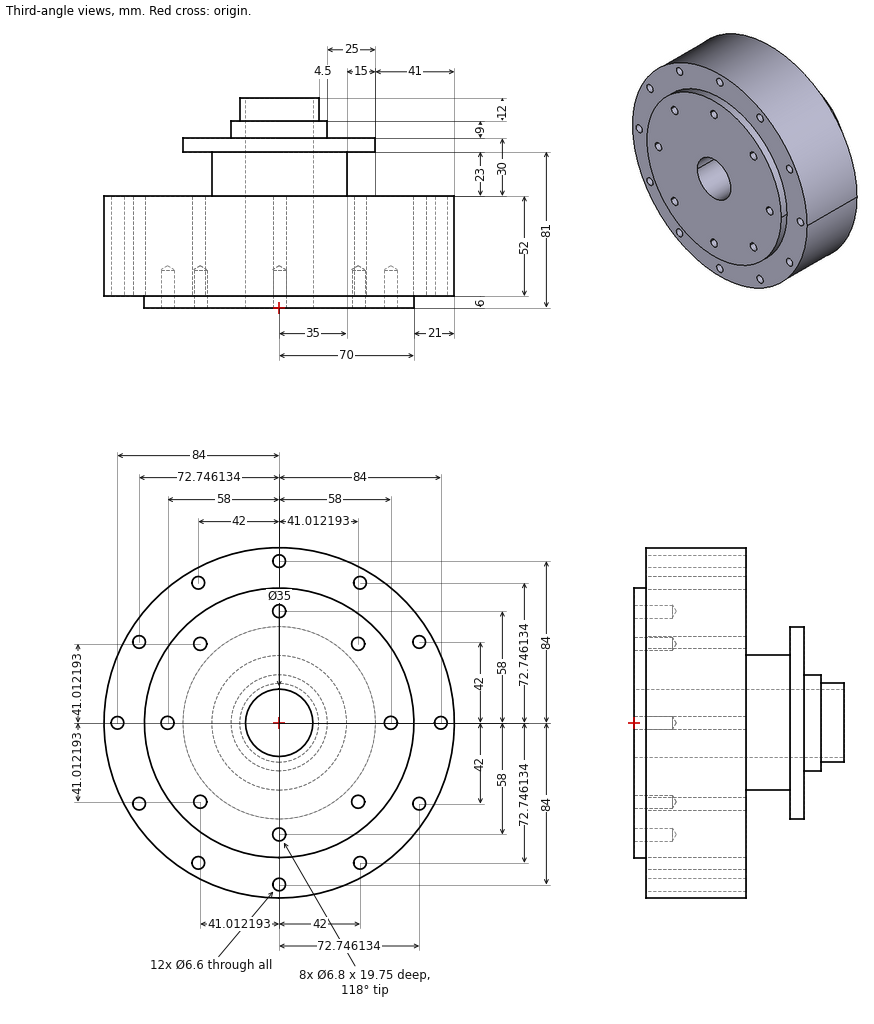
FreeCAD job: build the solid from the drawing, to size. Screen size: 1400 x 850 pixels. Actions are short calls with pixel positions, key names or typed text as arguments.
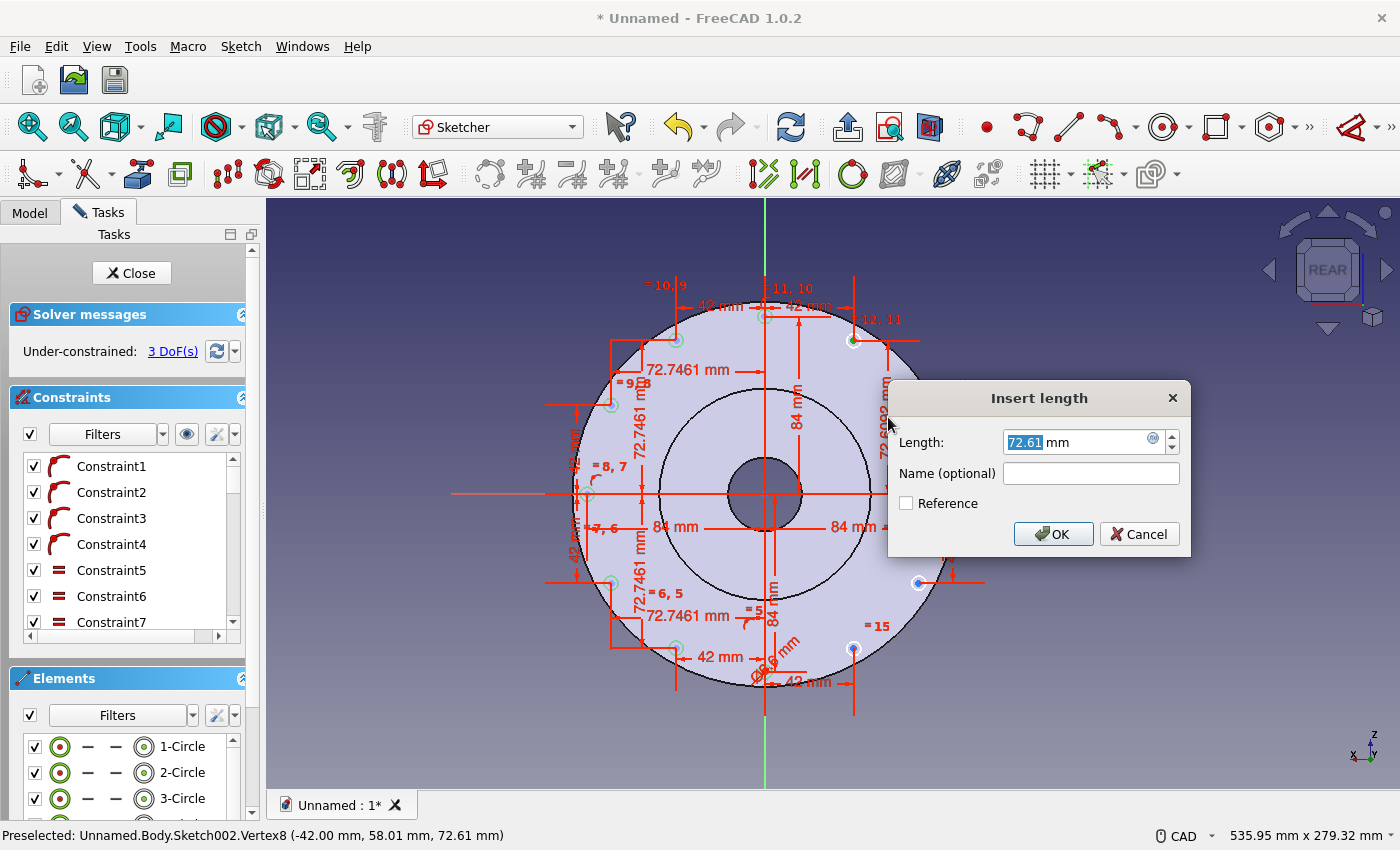
text(72.746134)
key(Return)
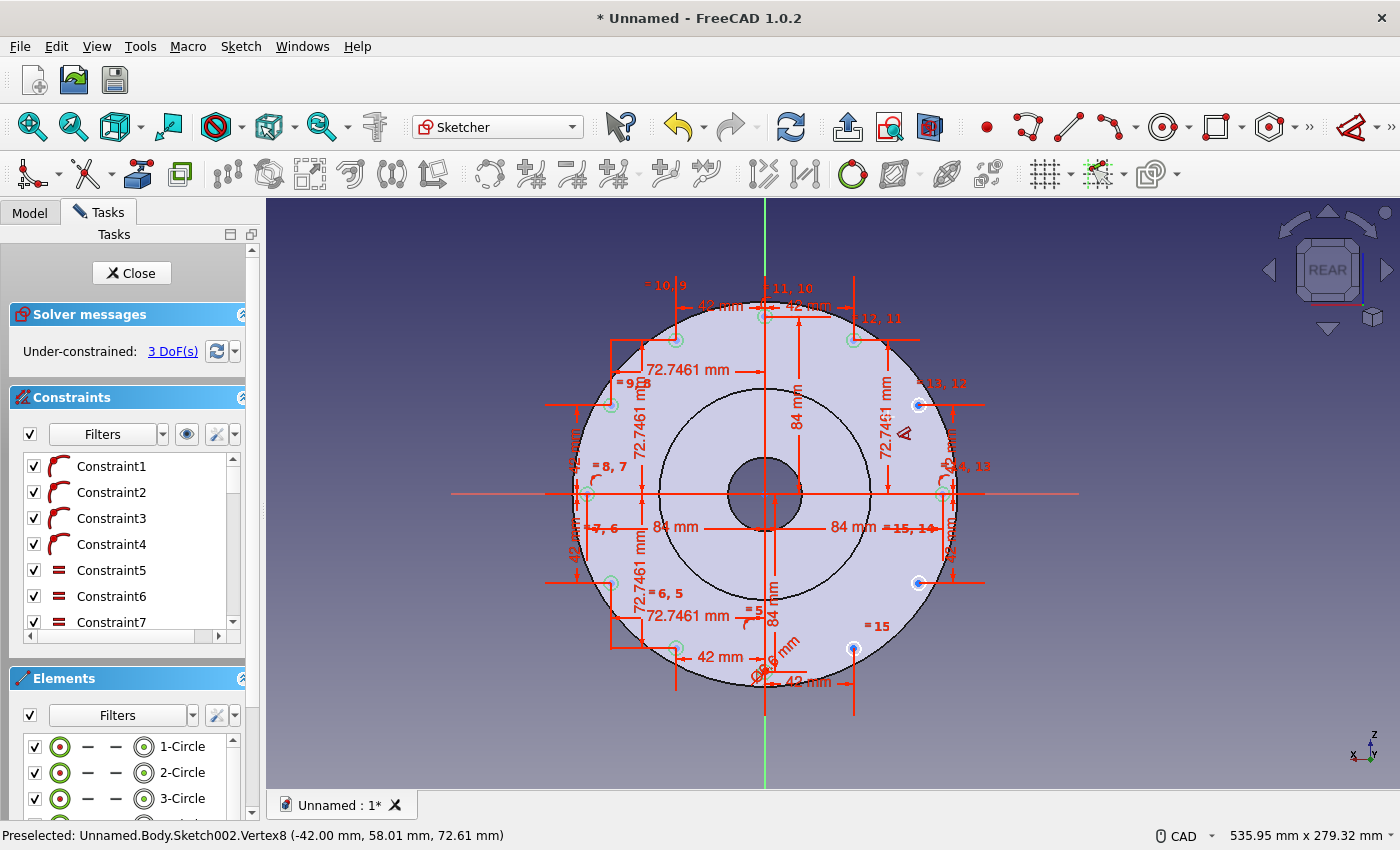
click(919, 405)
click(842, 371)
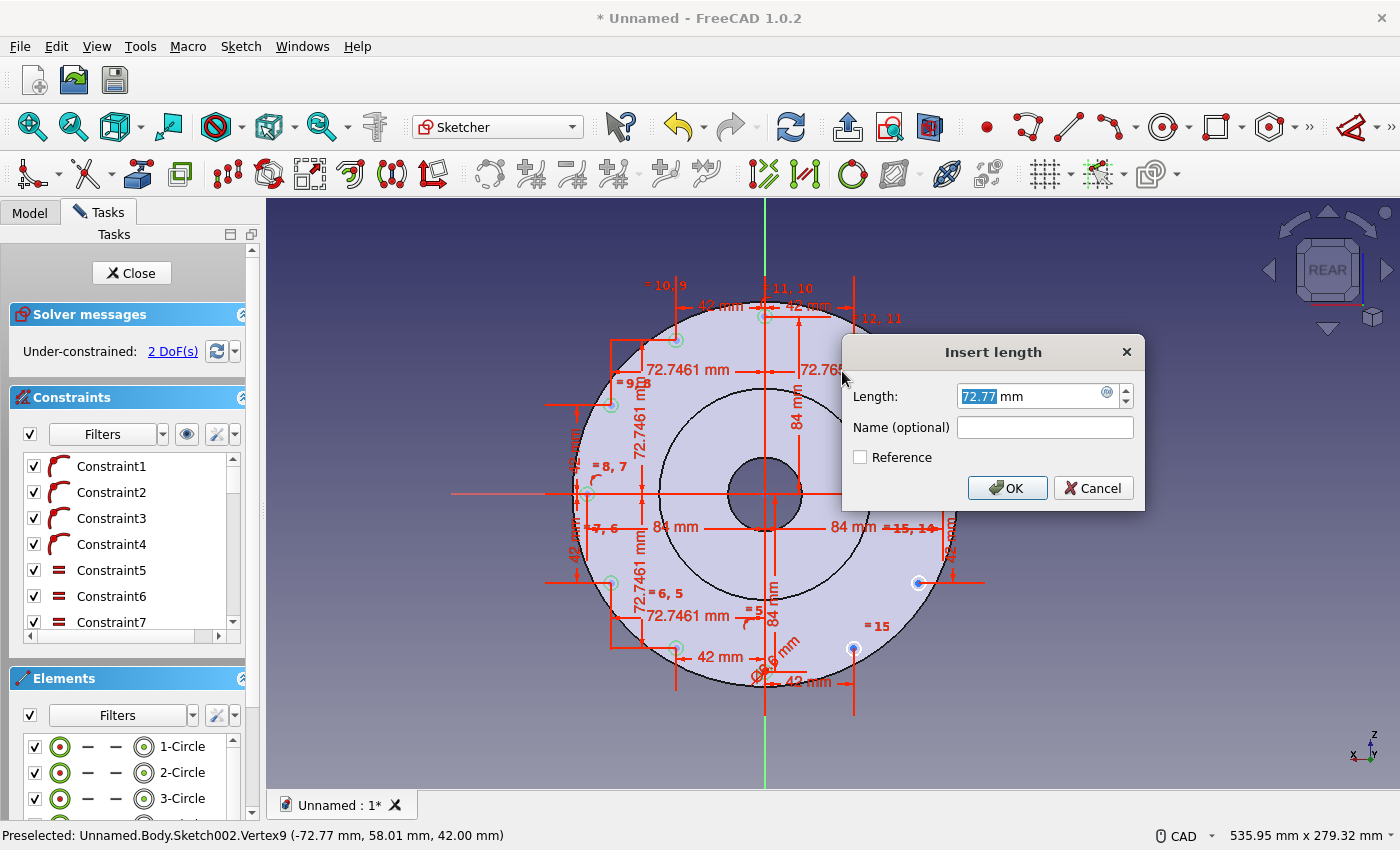
text(72.746134)
key(Return)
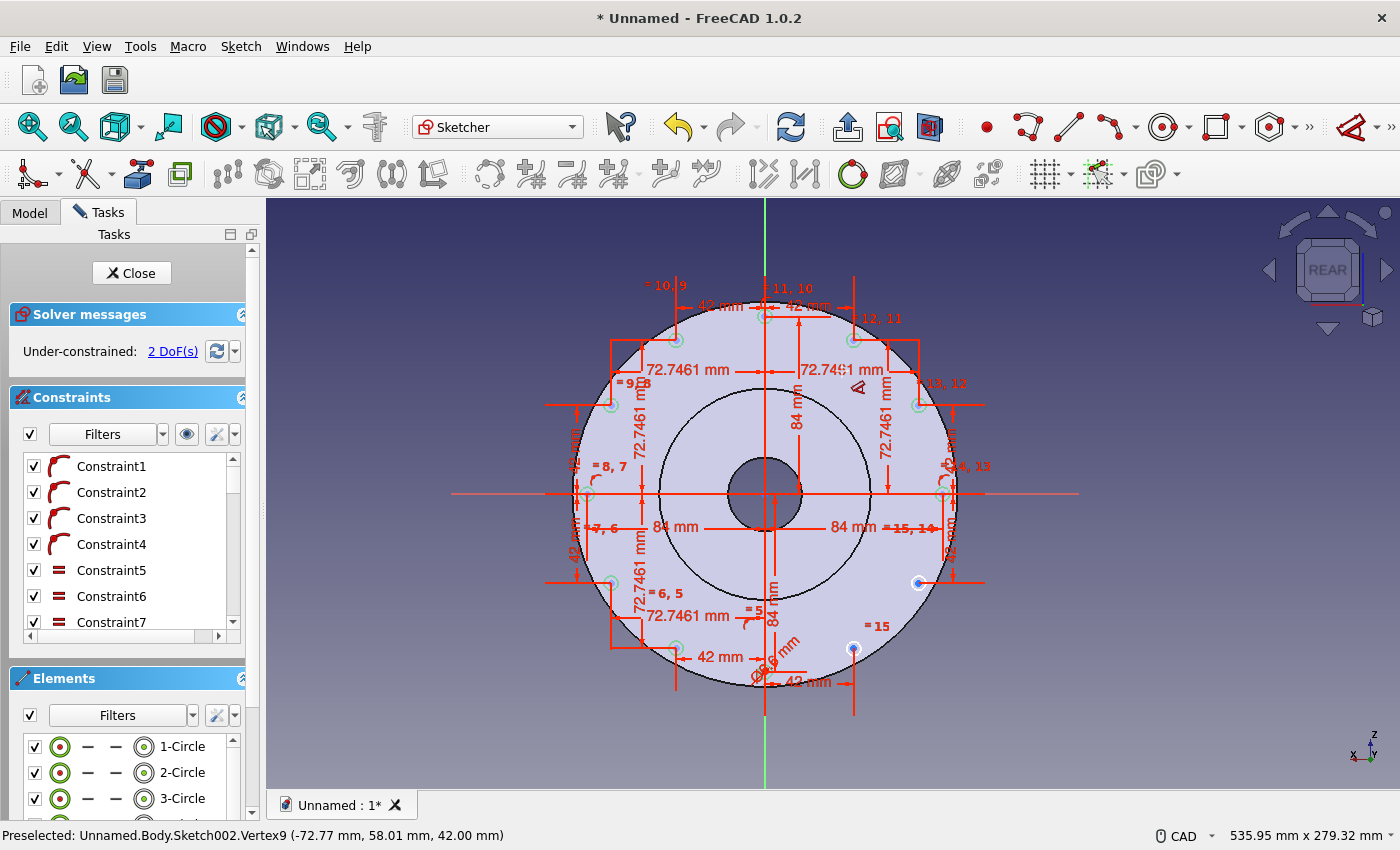
click(919, 583)
click(877, 617)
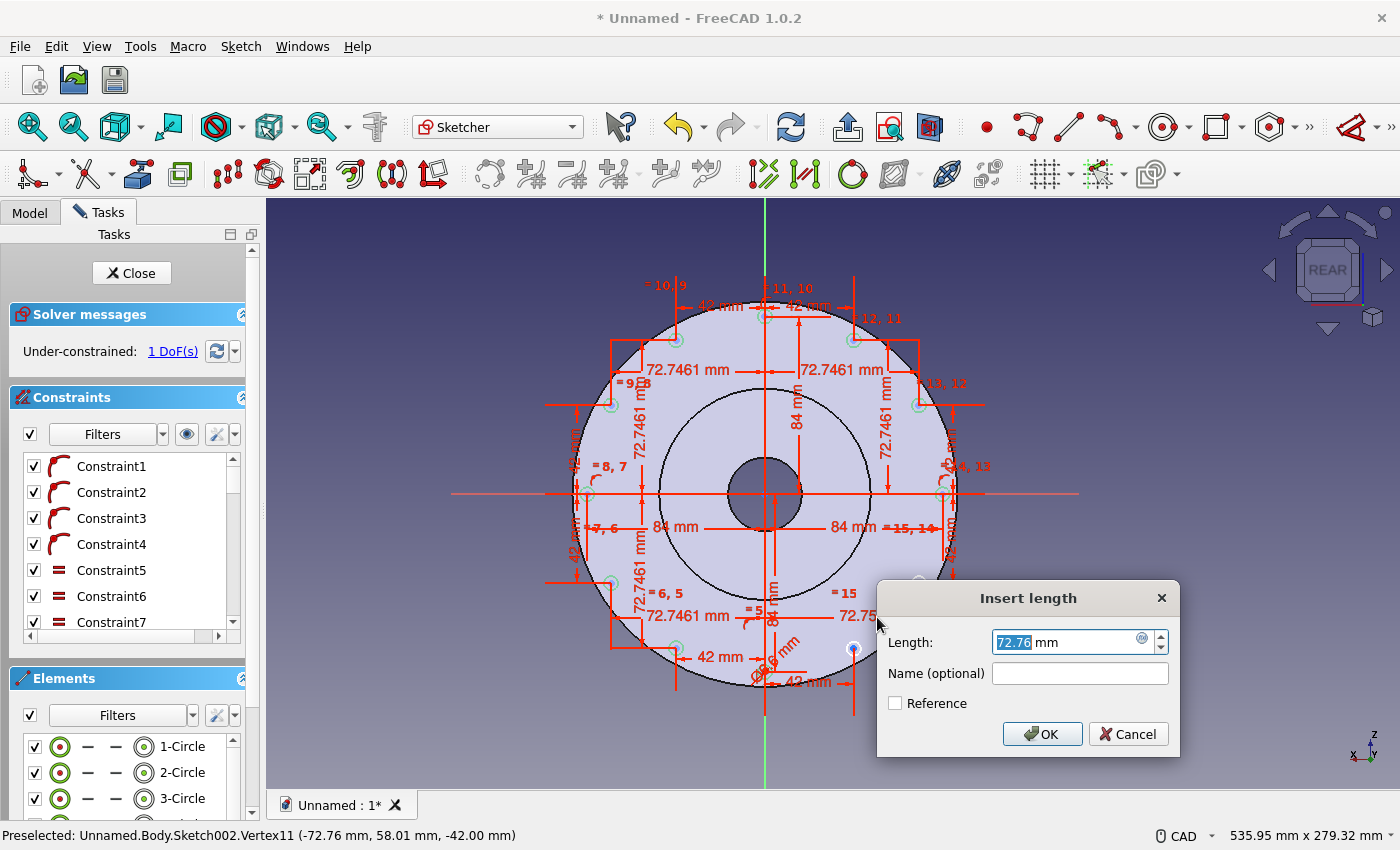
text(72.746134)
key(Return)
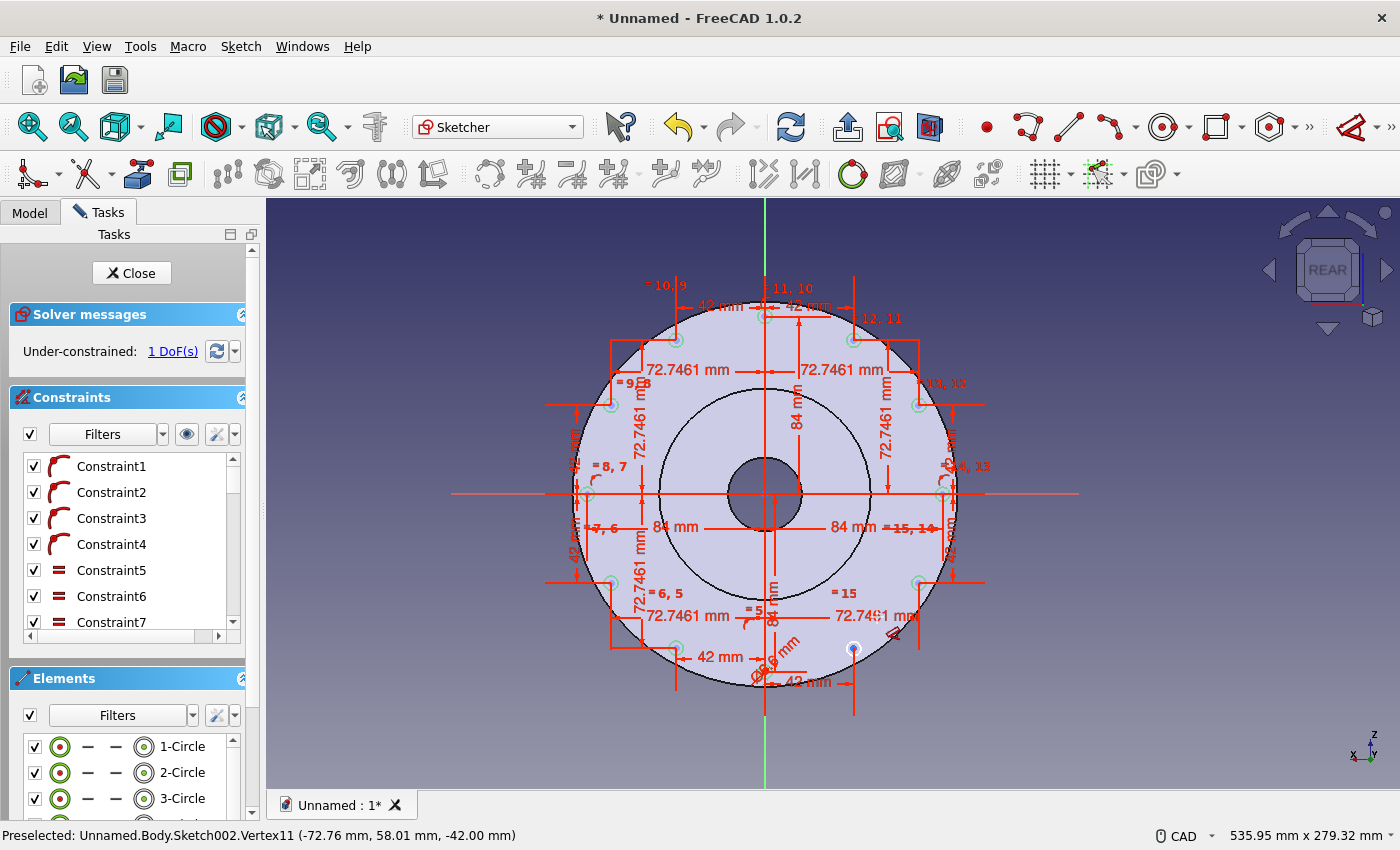
click(854, 649)
click(888, 571)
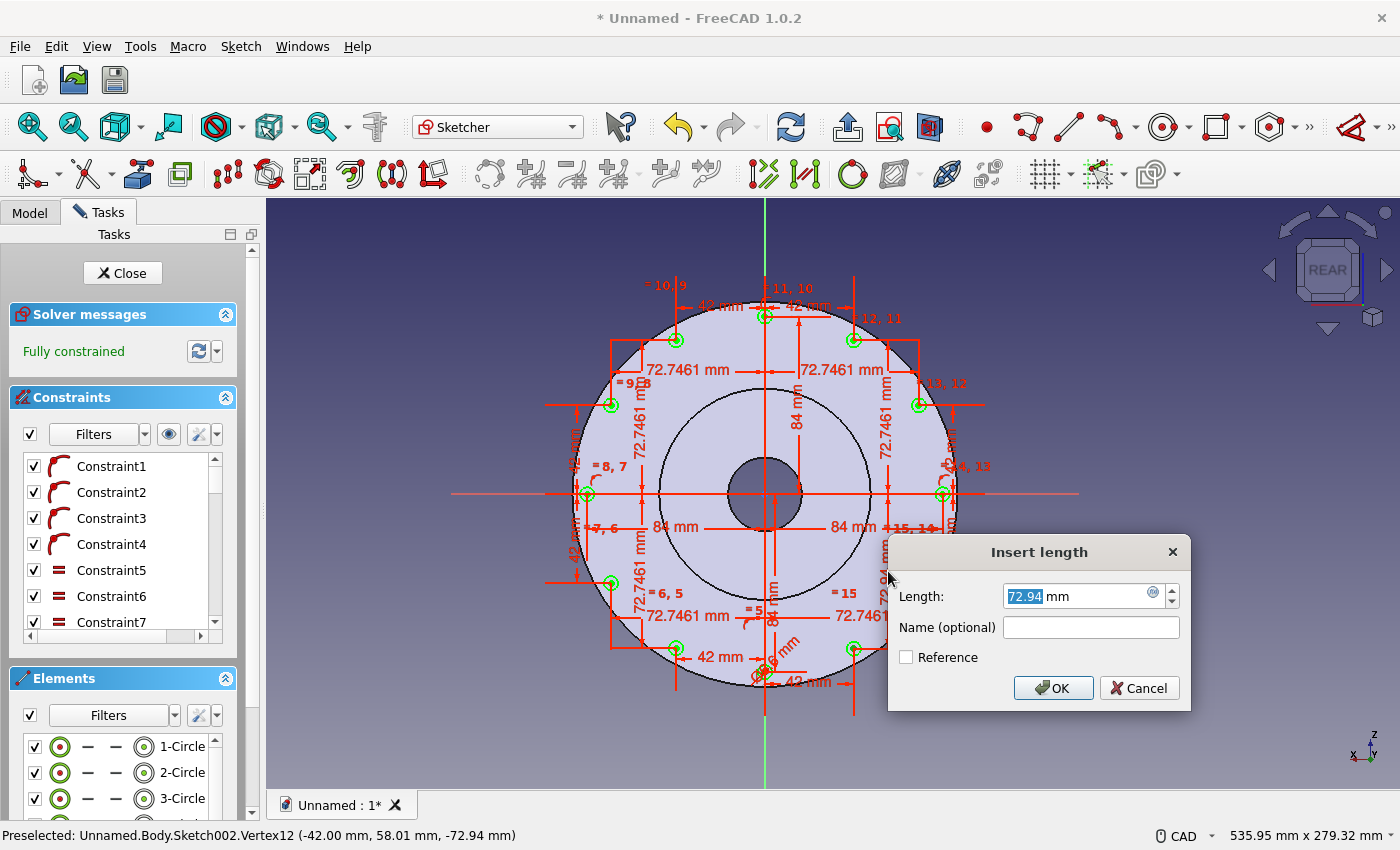
text(72.746134)
key(Return)
key(Escape)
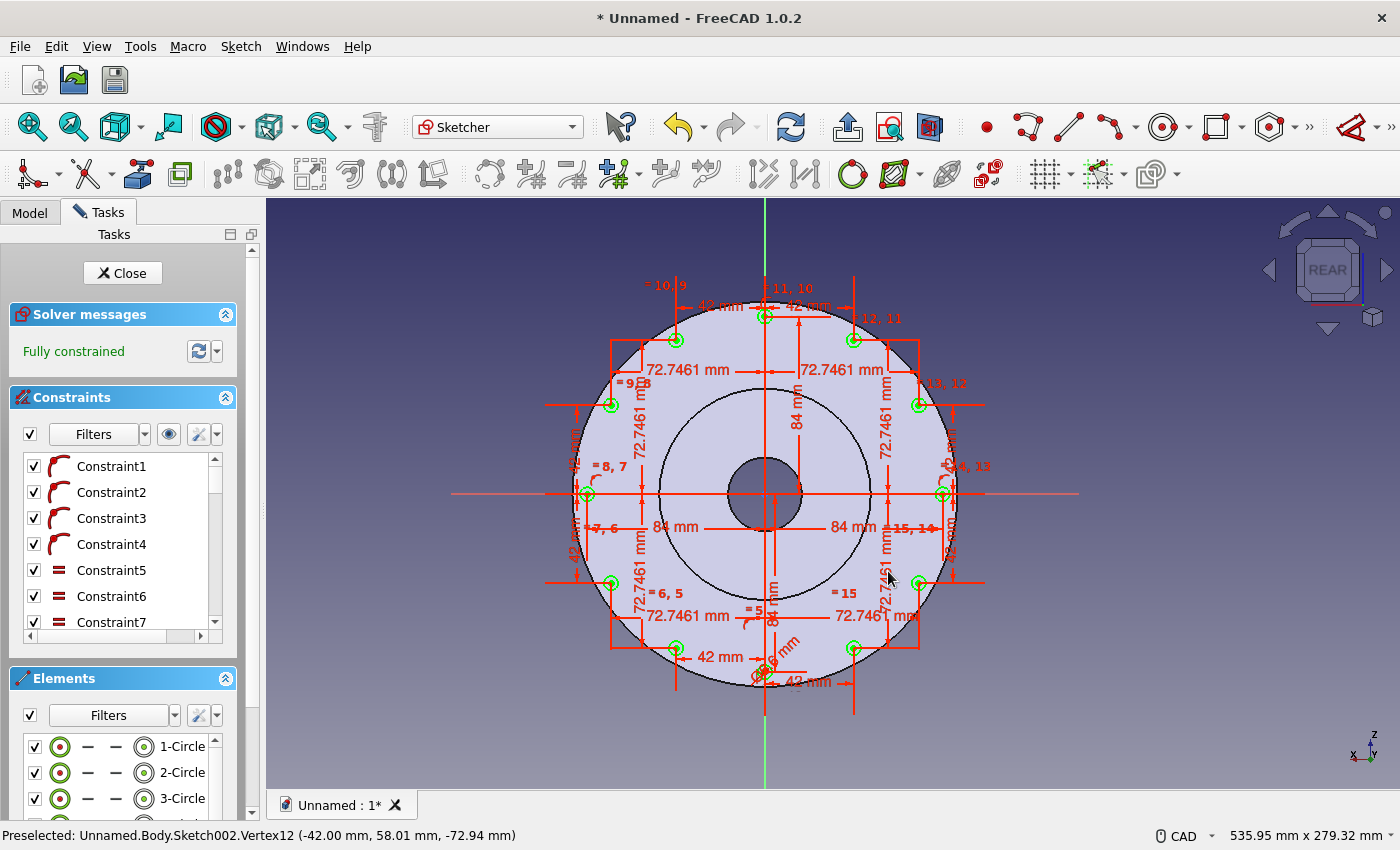
click(123, 273)